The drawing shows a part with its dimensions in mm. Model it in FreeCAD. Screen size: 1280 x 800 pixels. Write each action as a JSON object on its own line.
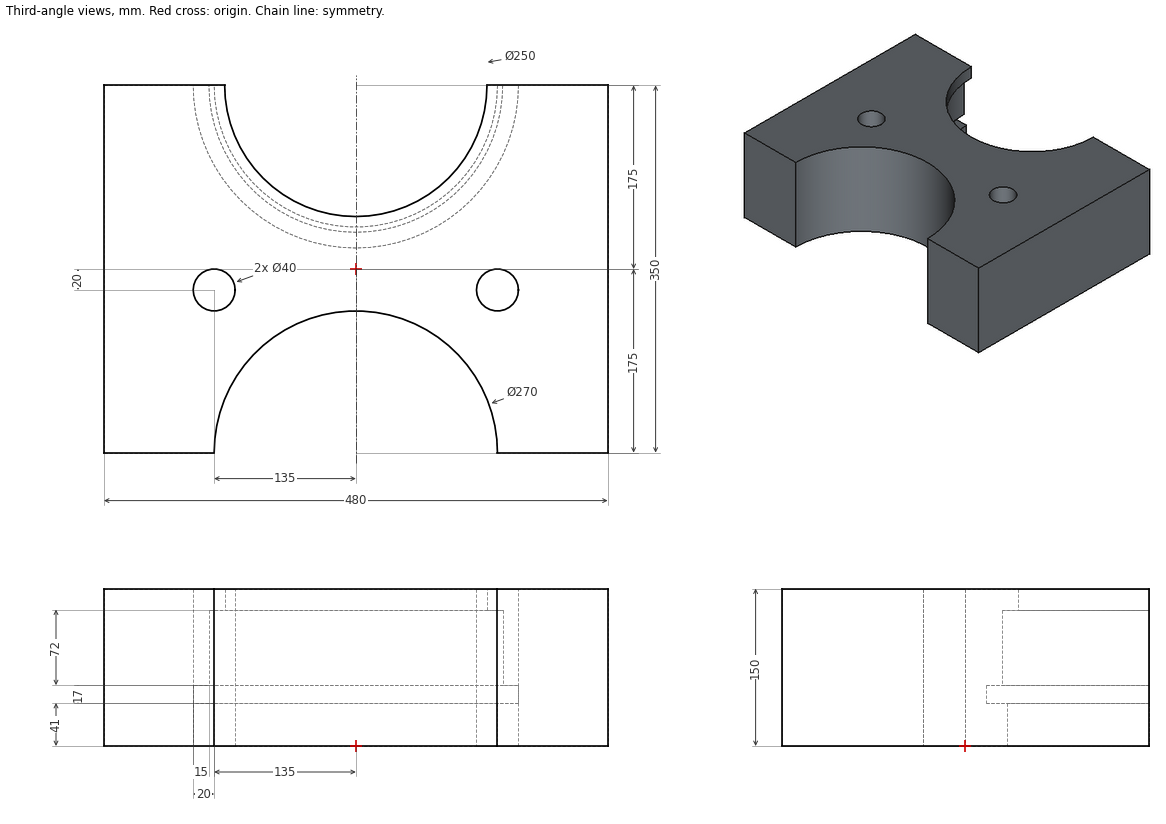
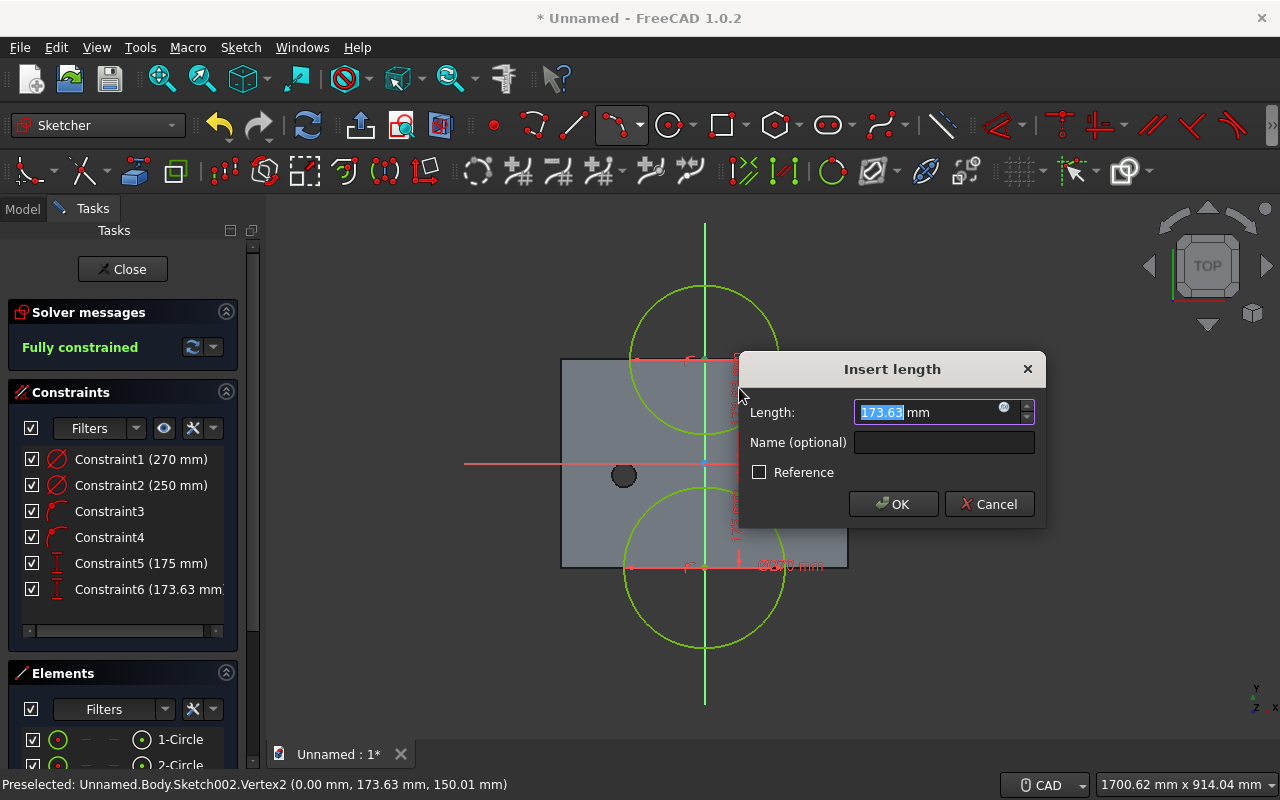
{"action": "type", "text": "175"}
{"action": "key", "text": "Return"}
{"action": "key", "text": "Escape"}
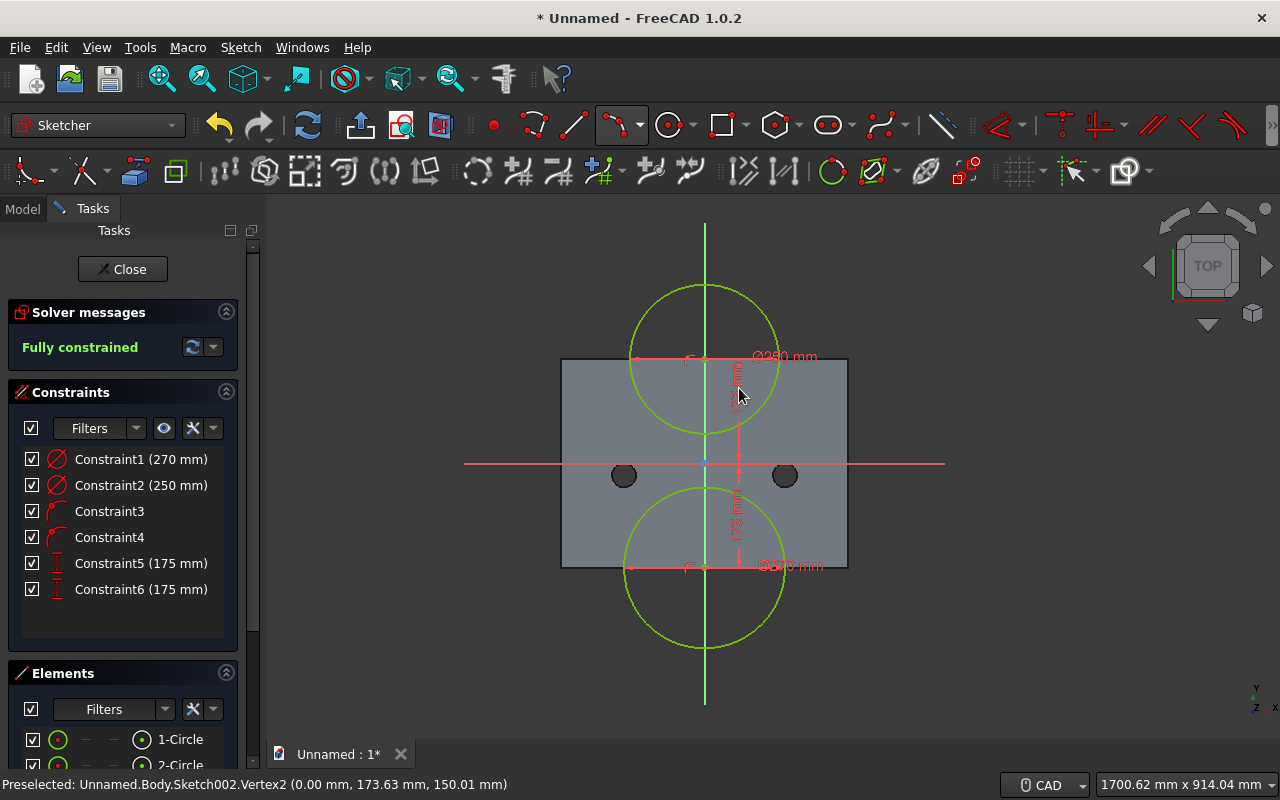
{"action": "left_click", "coordinate": [123, 269]}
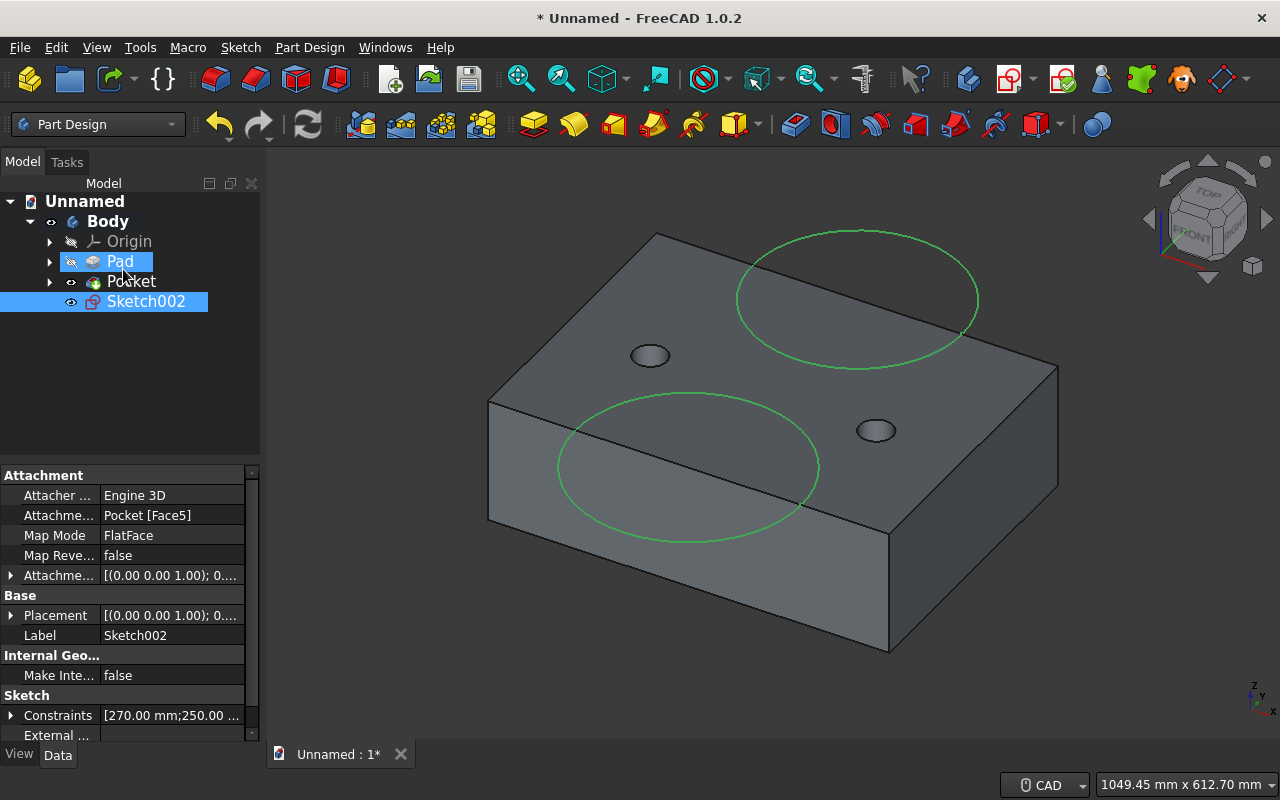
{"action": "left_click", "coordinate": [796, 124]}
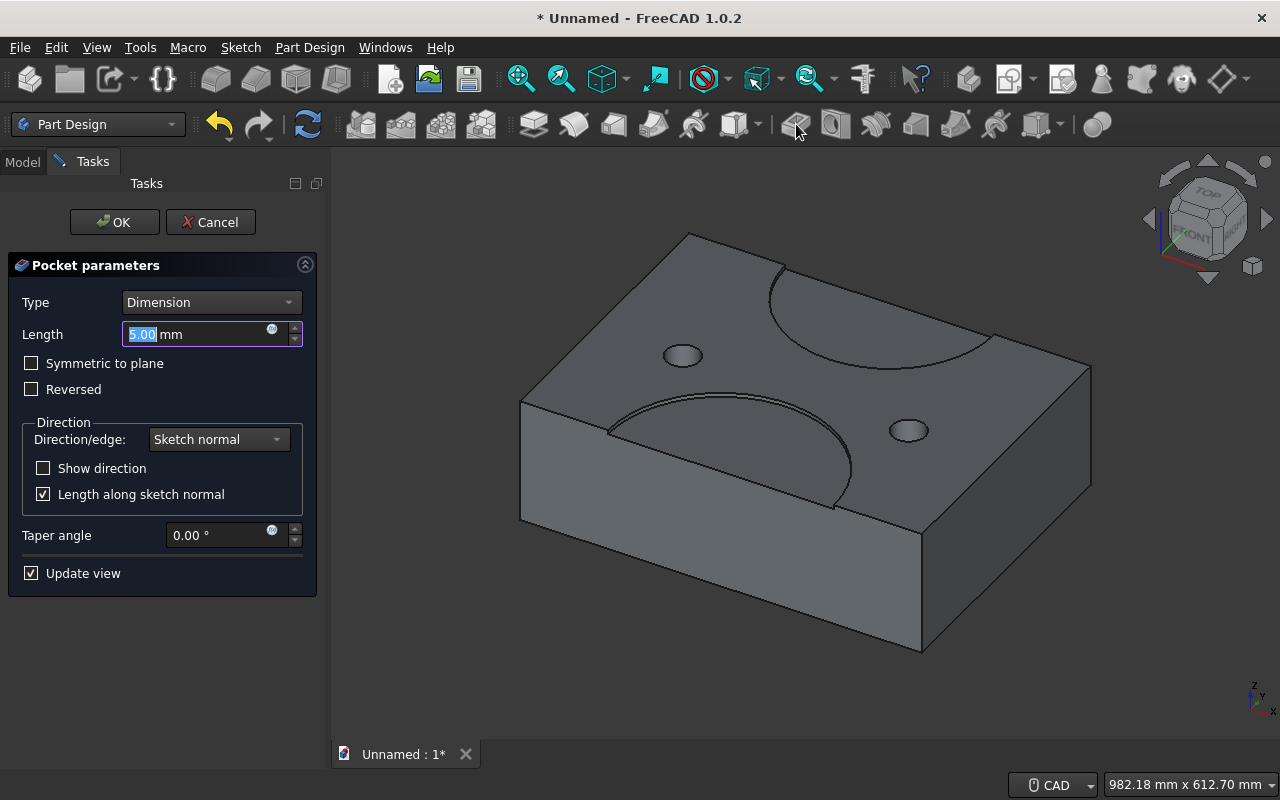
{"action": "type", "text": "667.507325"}
{"action": "key", "text": "Tab"}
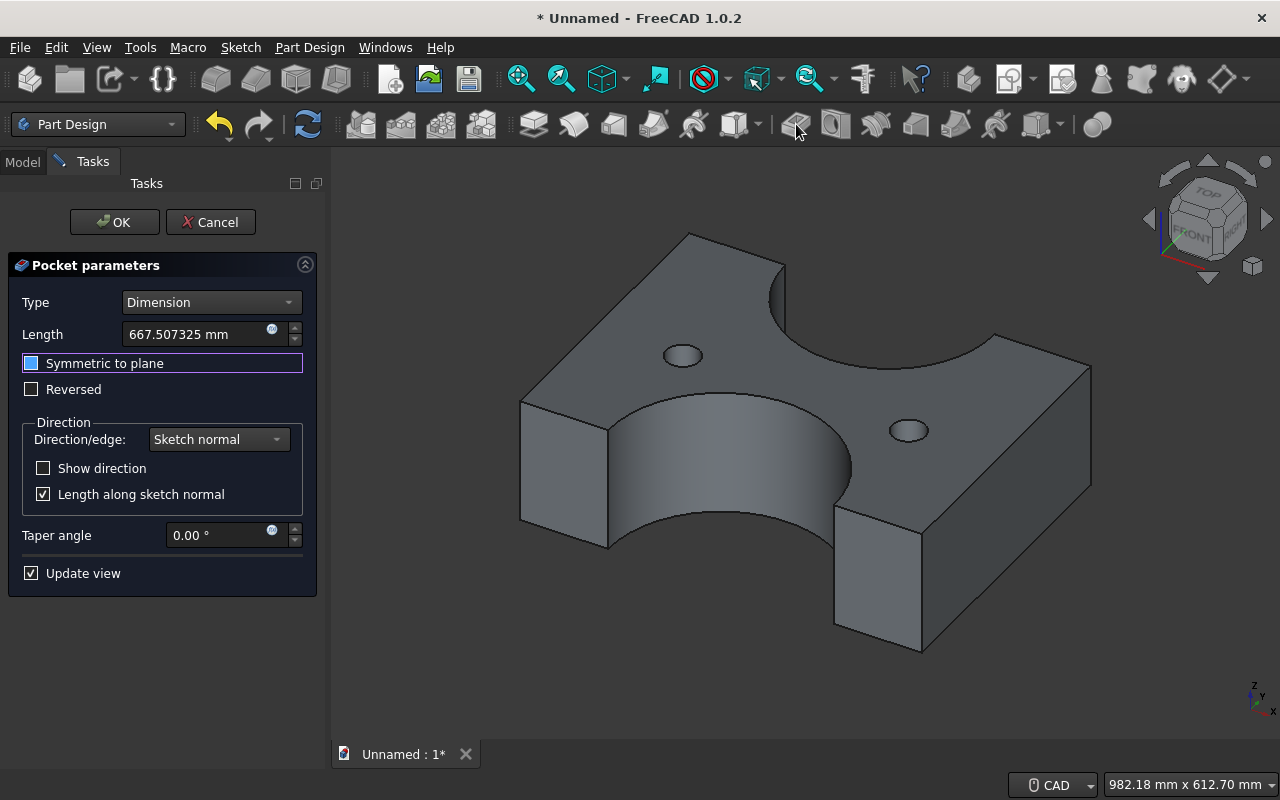
{"action": "left_click", "coordinate": [30, 363]}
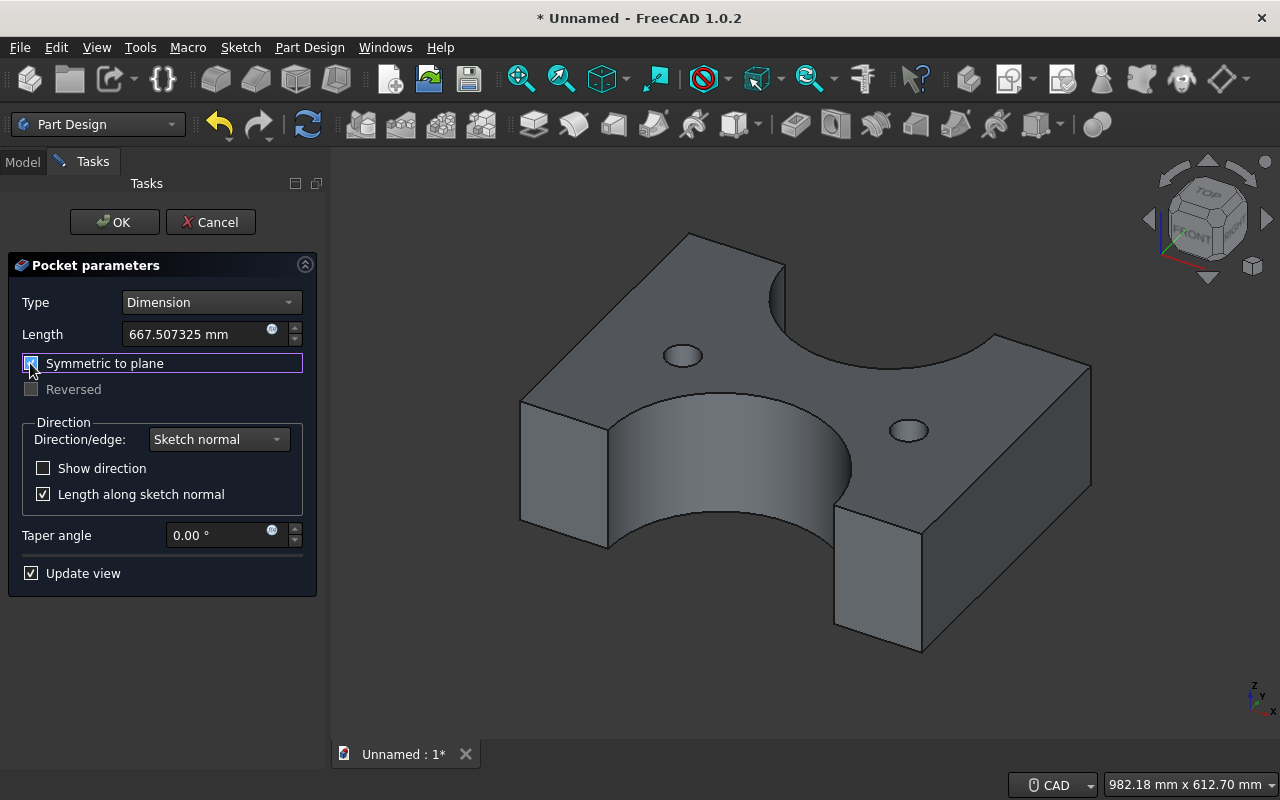
{"action": "left_click", "coordinate": [115, 222]}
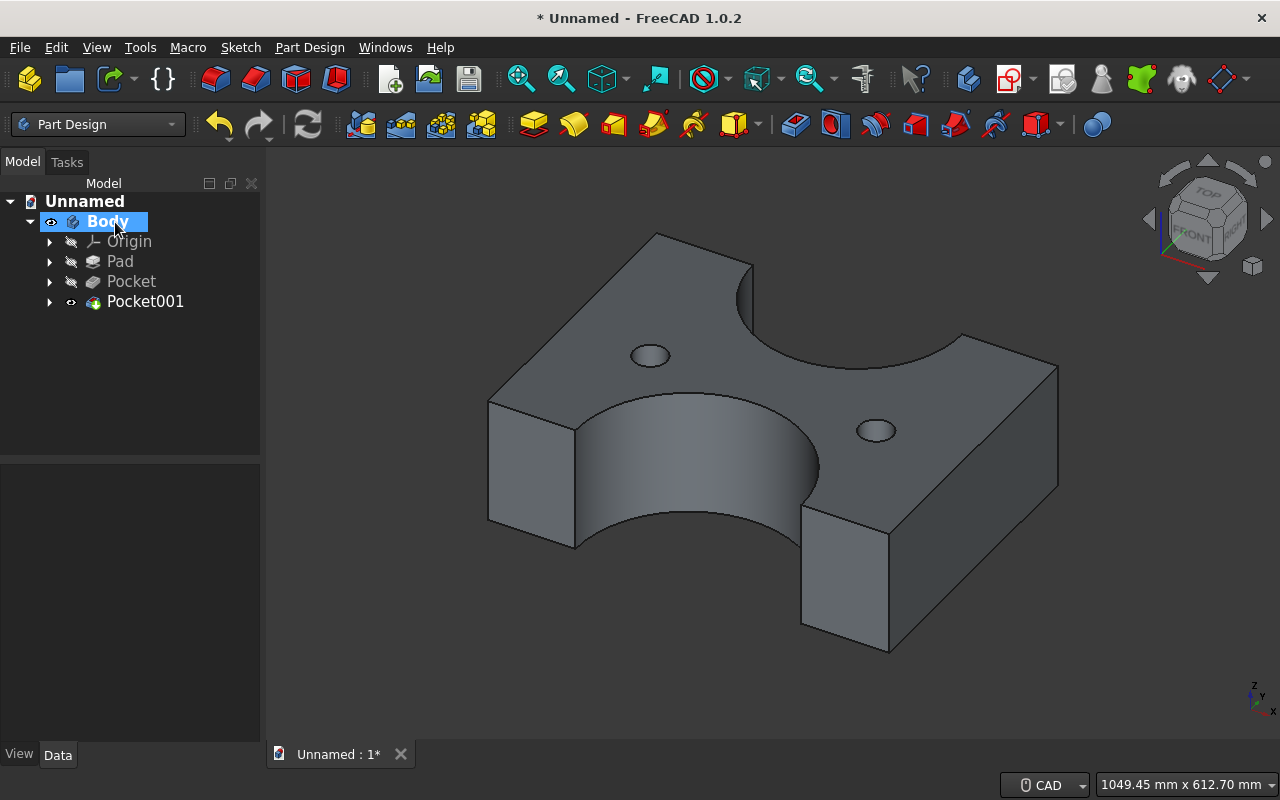
{"action": "key", "text": "4"}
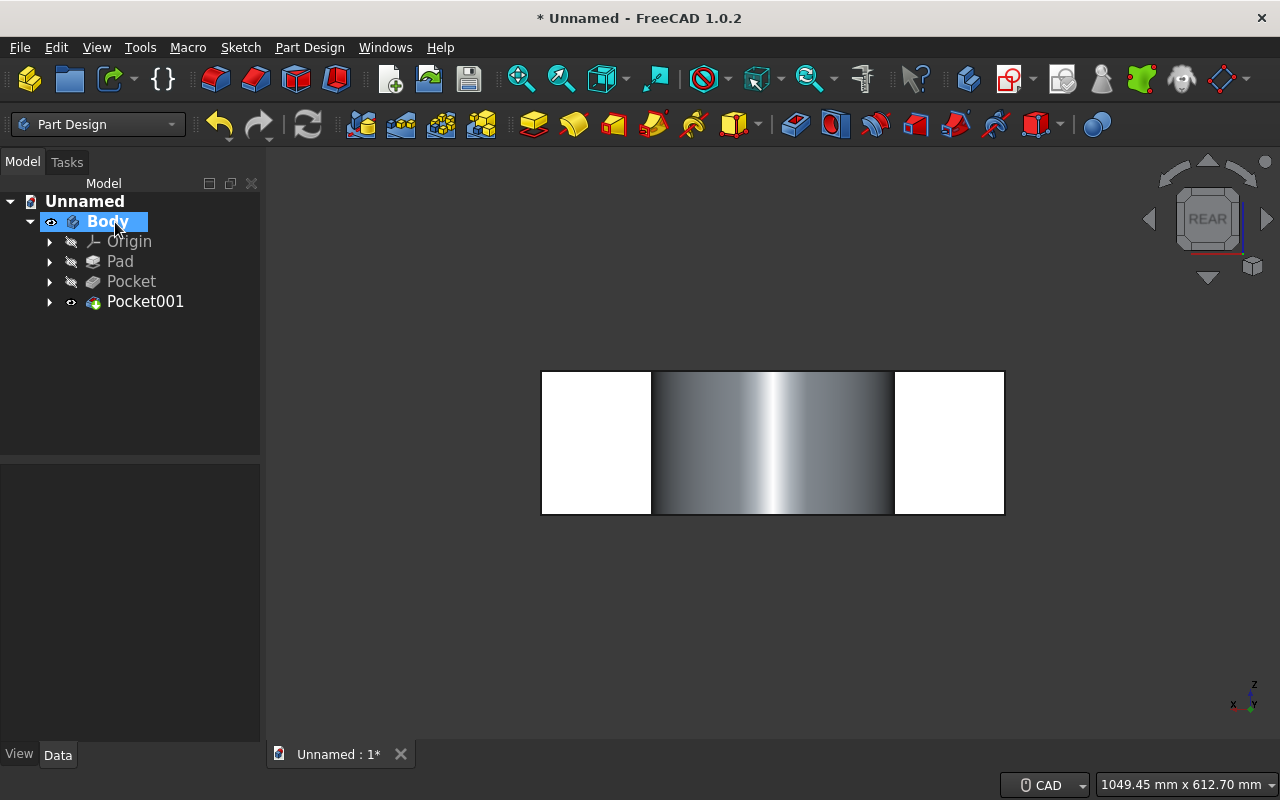
{"action": "left_click", "coordinate": [597, 442]}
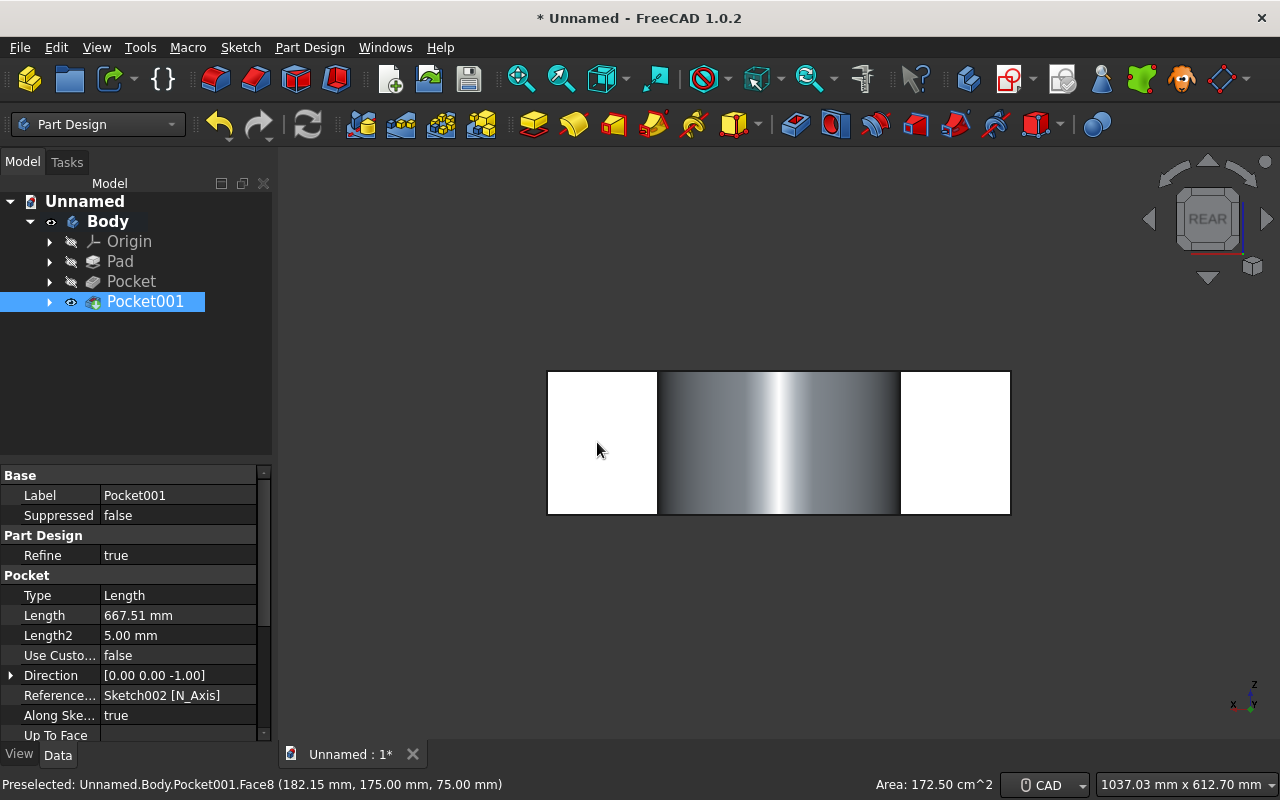
{"action": "left_click", "coordinate": [1010, 80]}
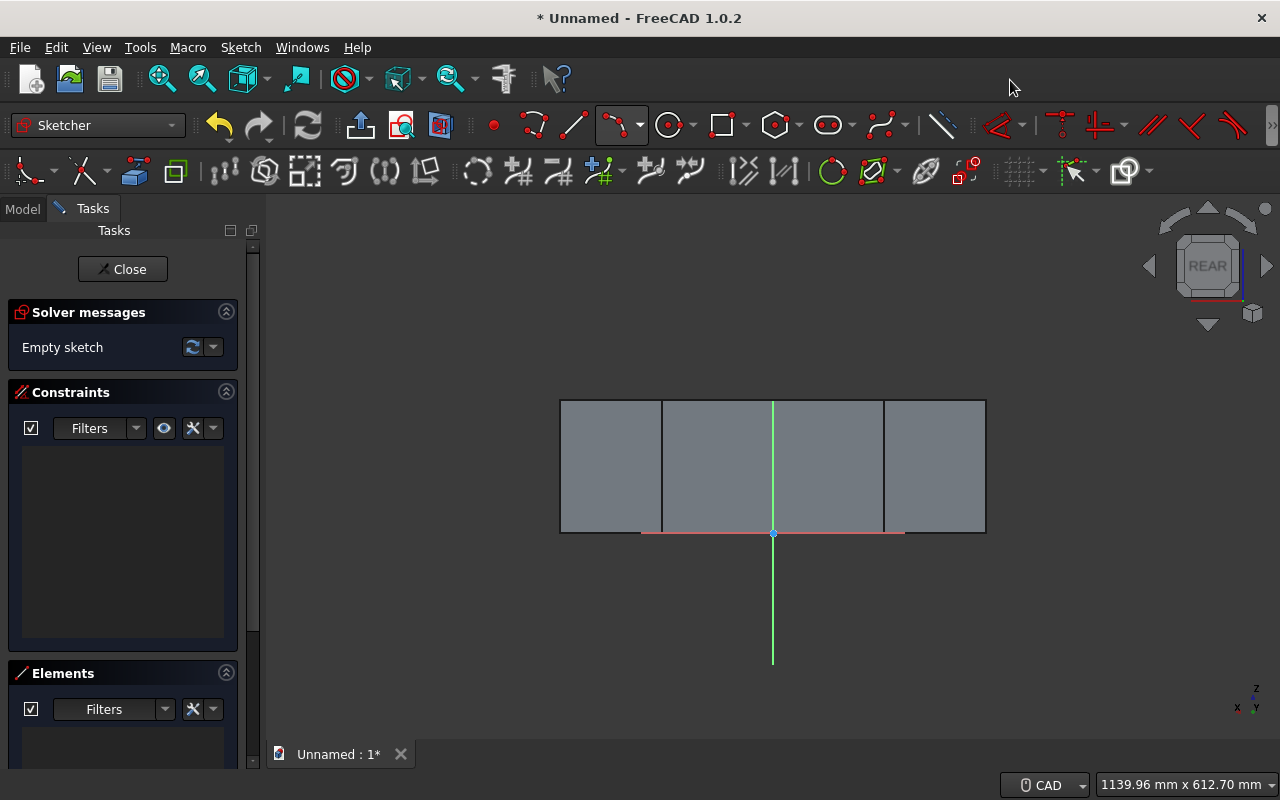
{"action": "scroll", "coordinate": [922, 481], "scroll_direction": "up", "scroll_amount": 5}